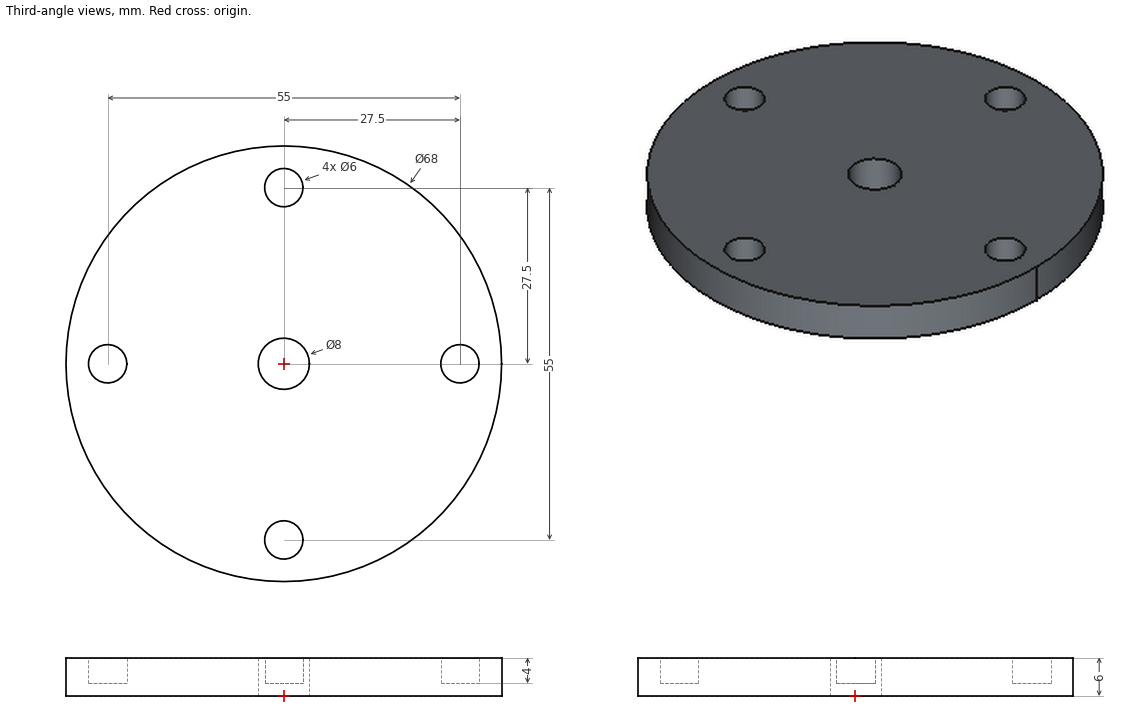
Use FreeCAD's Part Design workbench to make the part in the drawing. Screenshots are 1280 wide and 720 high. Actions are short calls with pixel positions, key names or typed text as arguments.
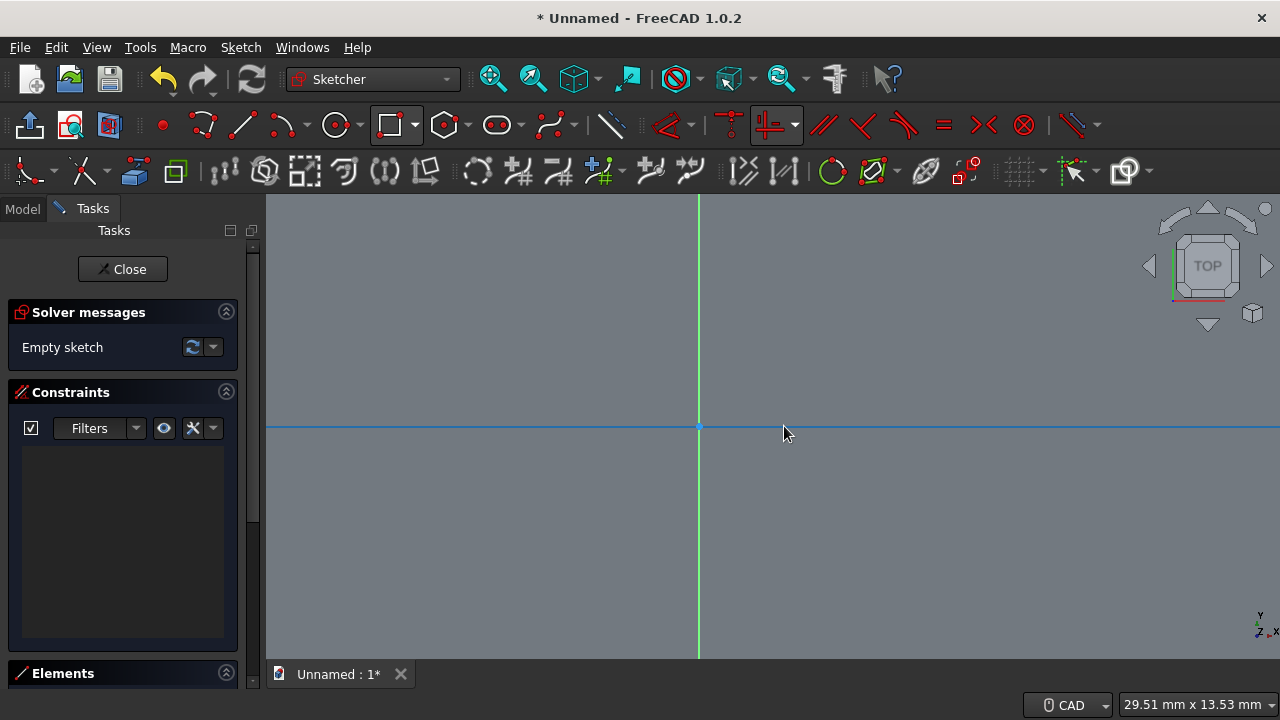
key(g)
key(c)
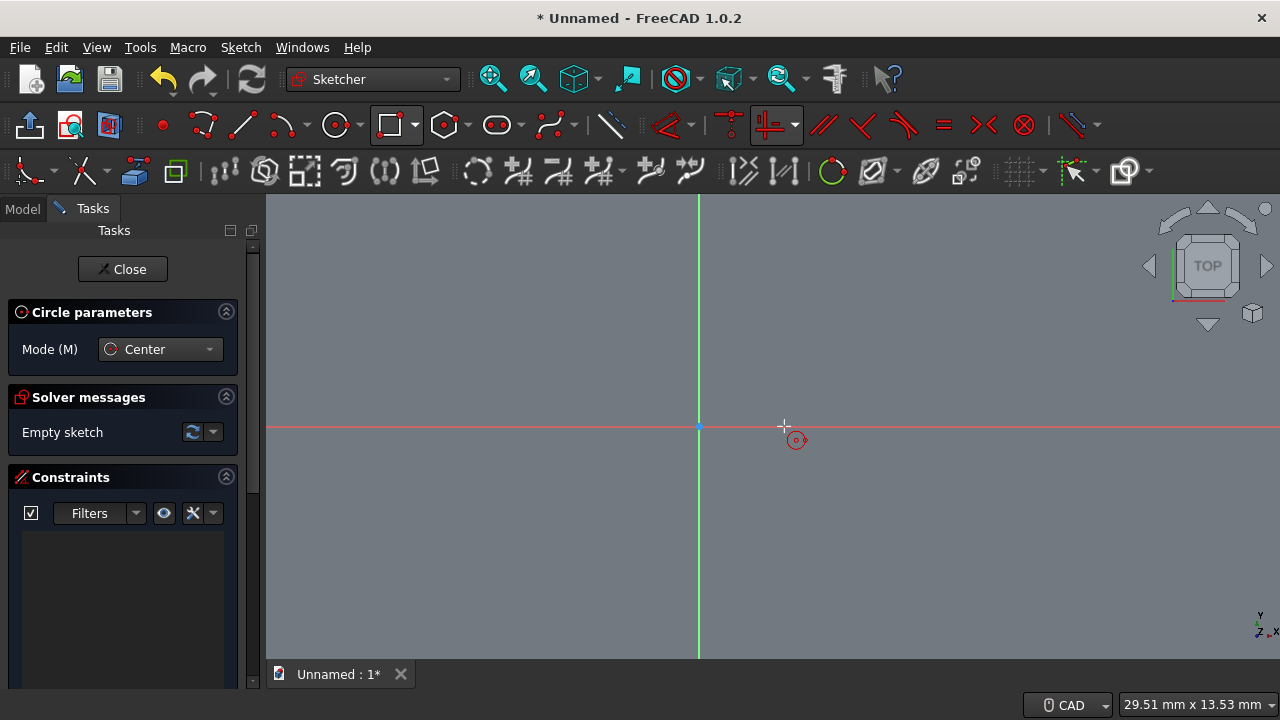
click(699, 426)
click(797, 329)
key(Escape)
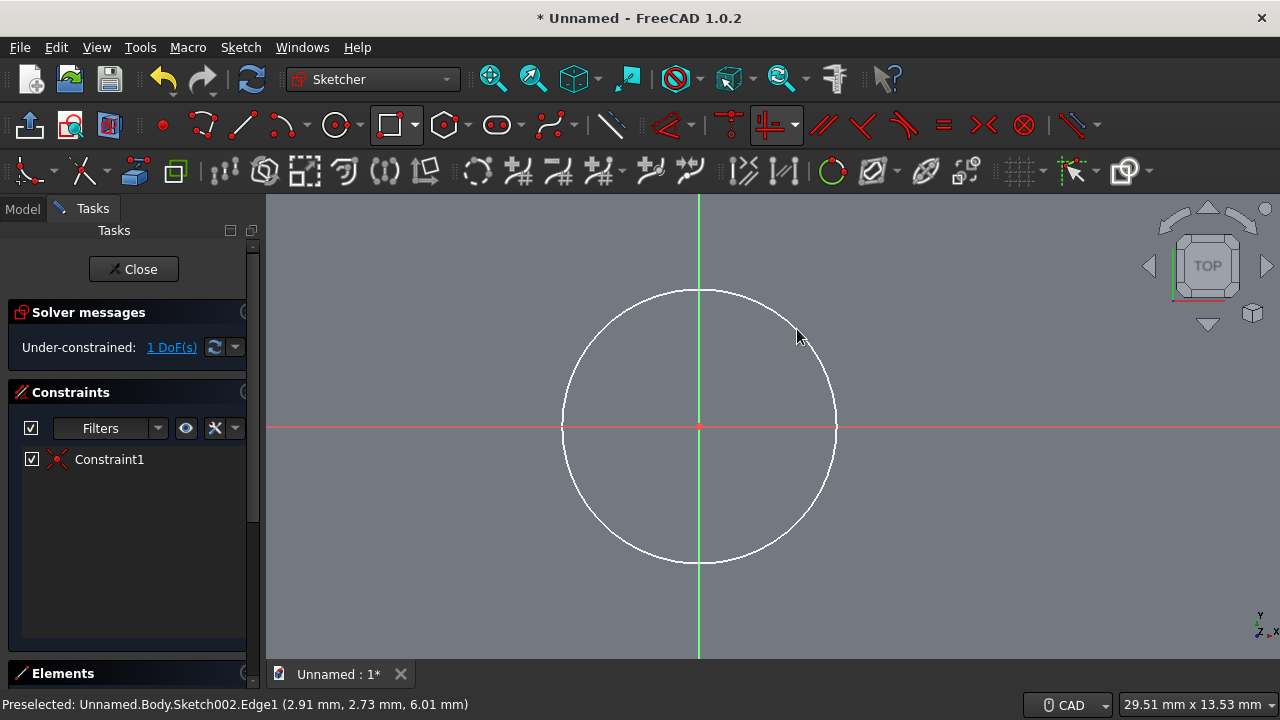
key(d)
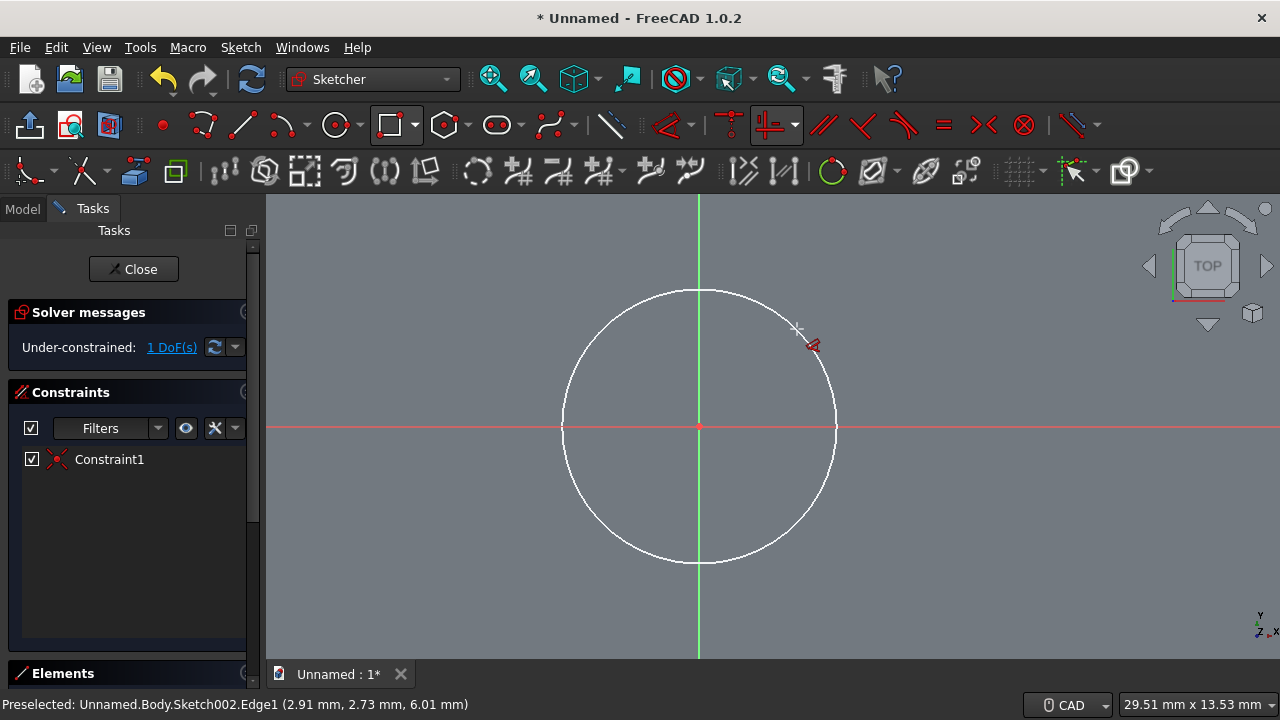
click(796, 329)
click(819, 306)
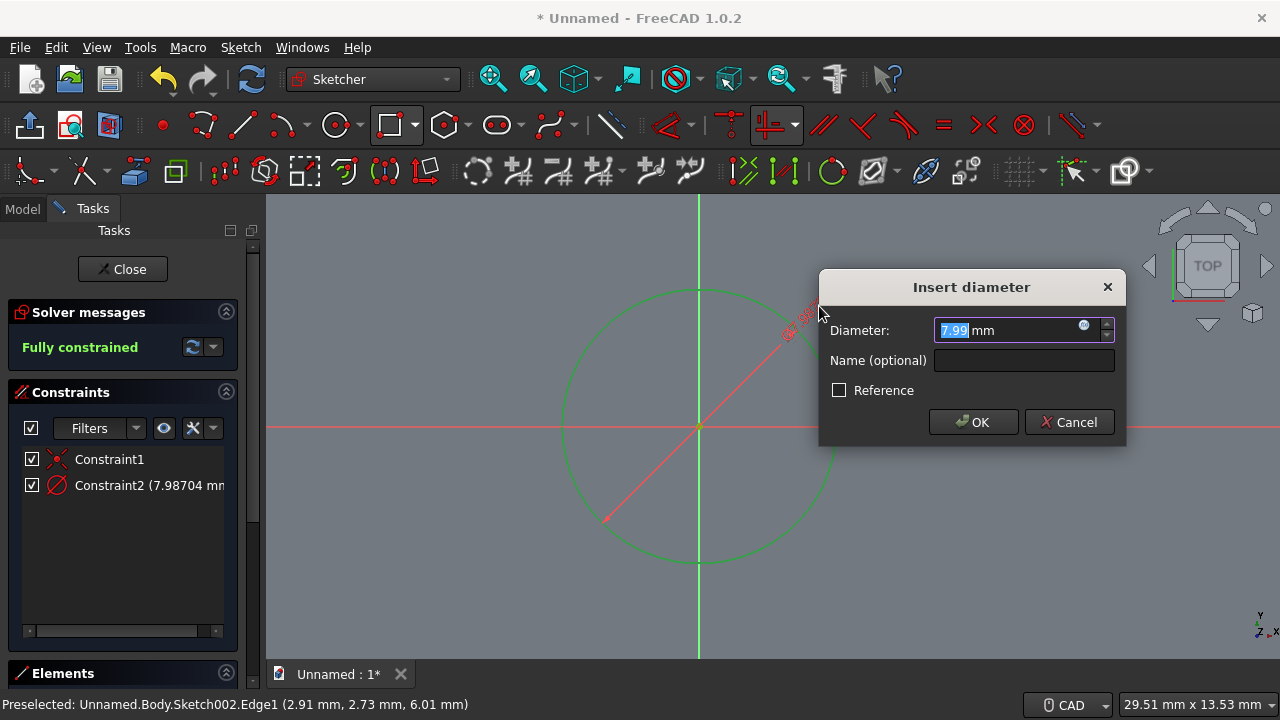
text(8)
key(Return)
key(Escape)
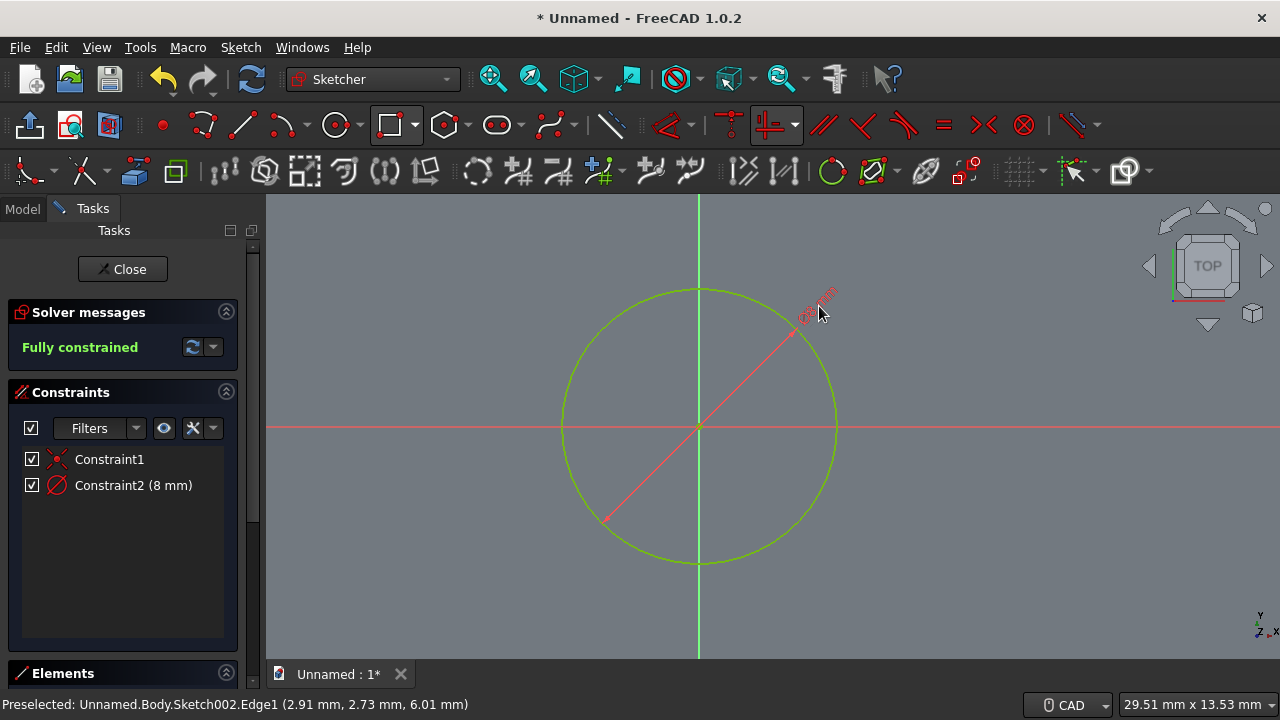
click(123, 269)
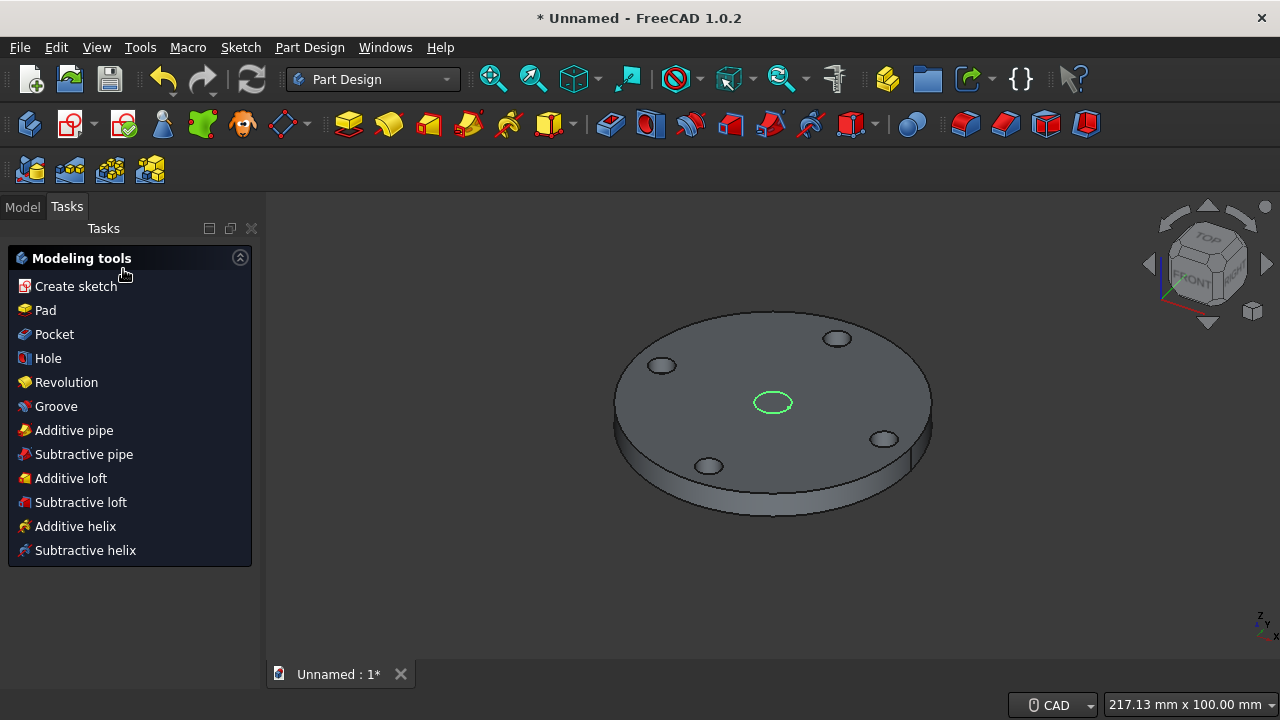
click(612, 124)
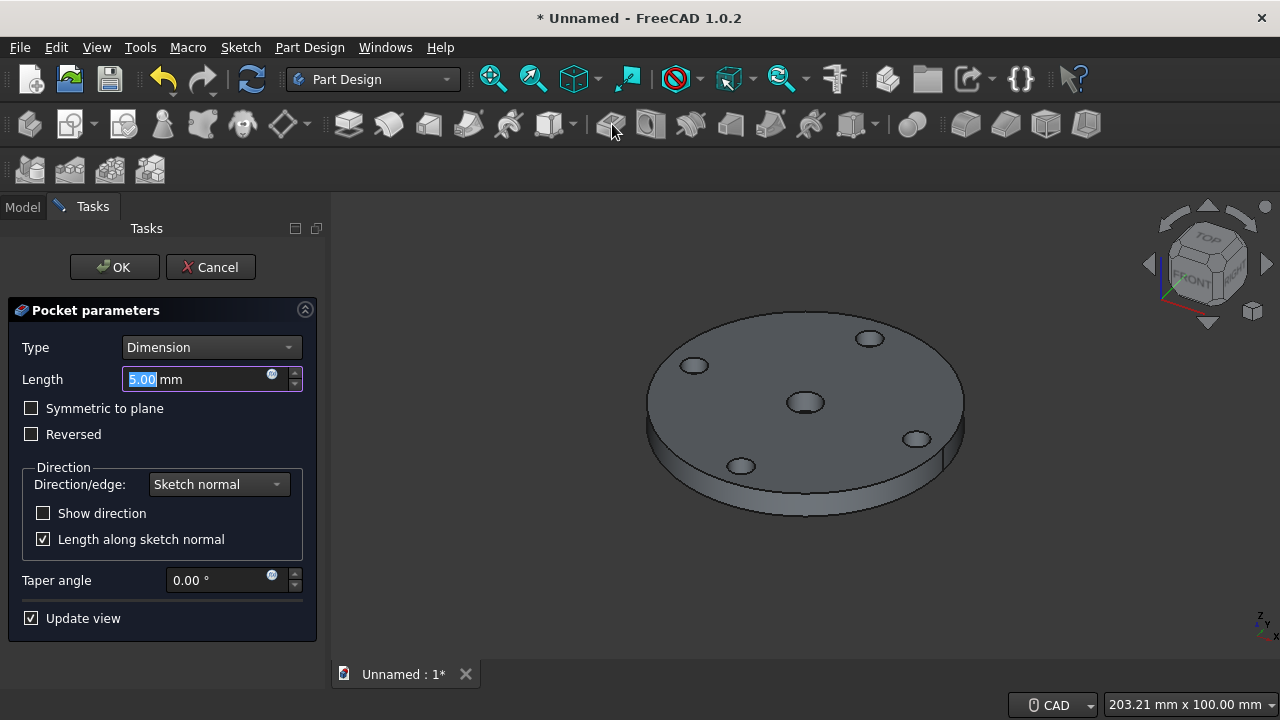
click(212, 348)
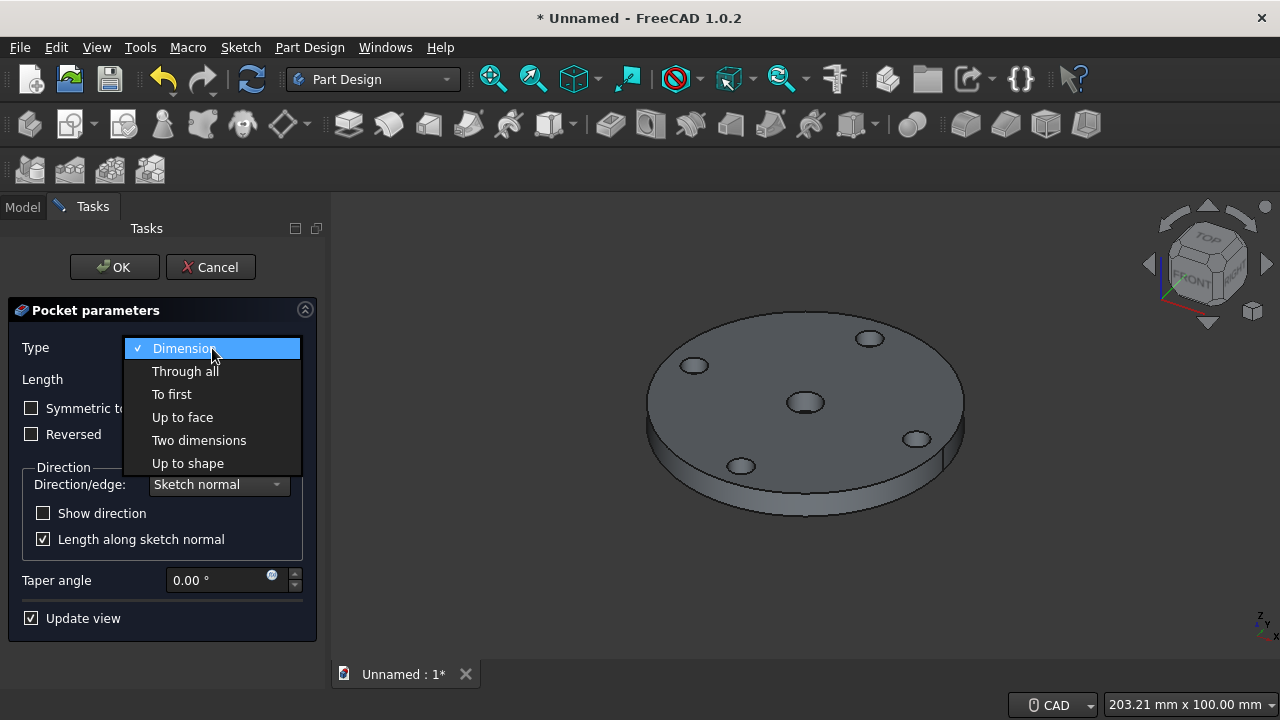
click(212, 372)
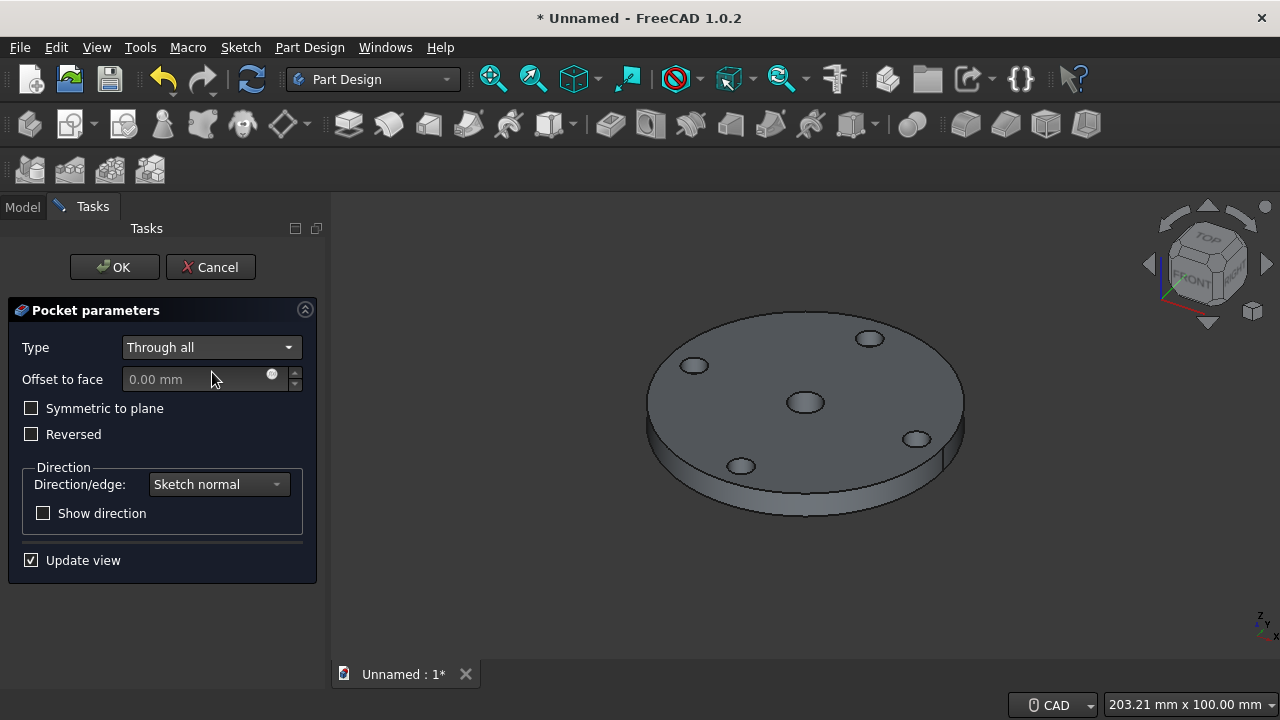
click(115, 267)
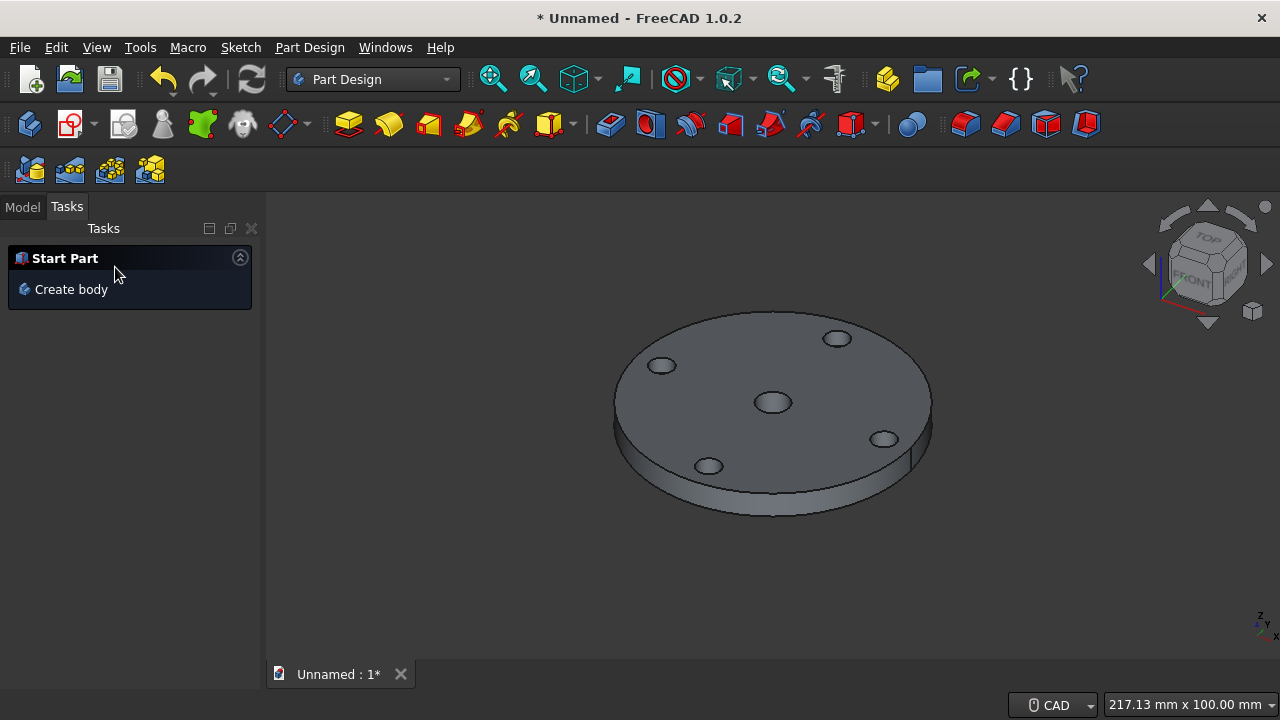
key(0)